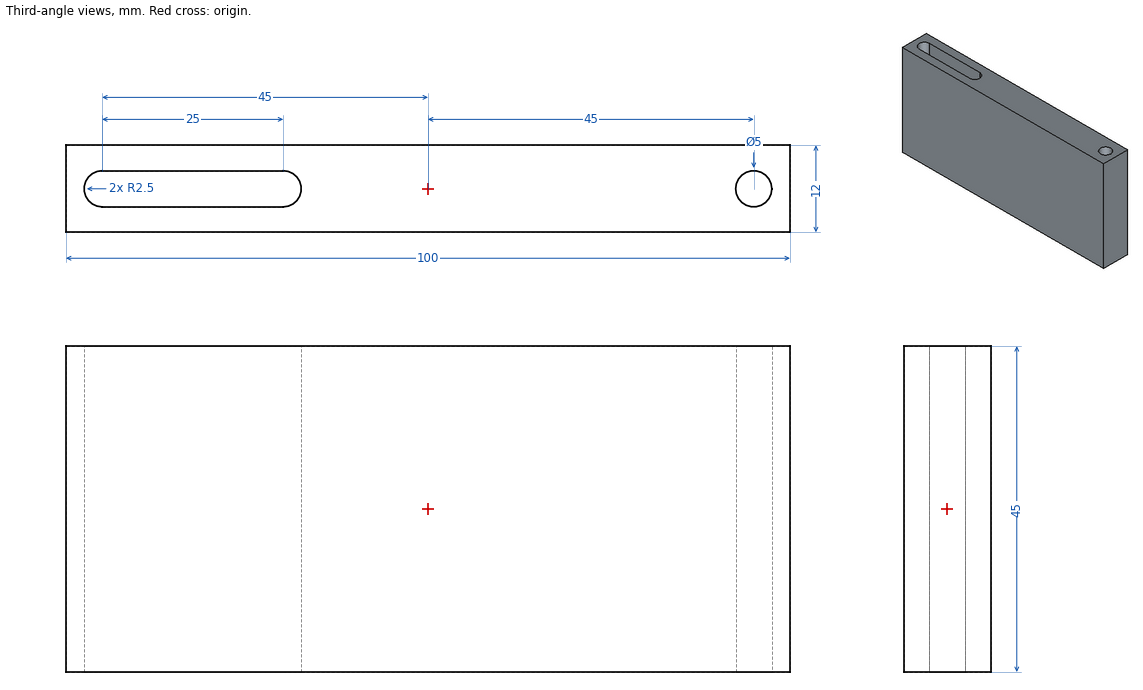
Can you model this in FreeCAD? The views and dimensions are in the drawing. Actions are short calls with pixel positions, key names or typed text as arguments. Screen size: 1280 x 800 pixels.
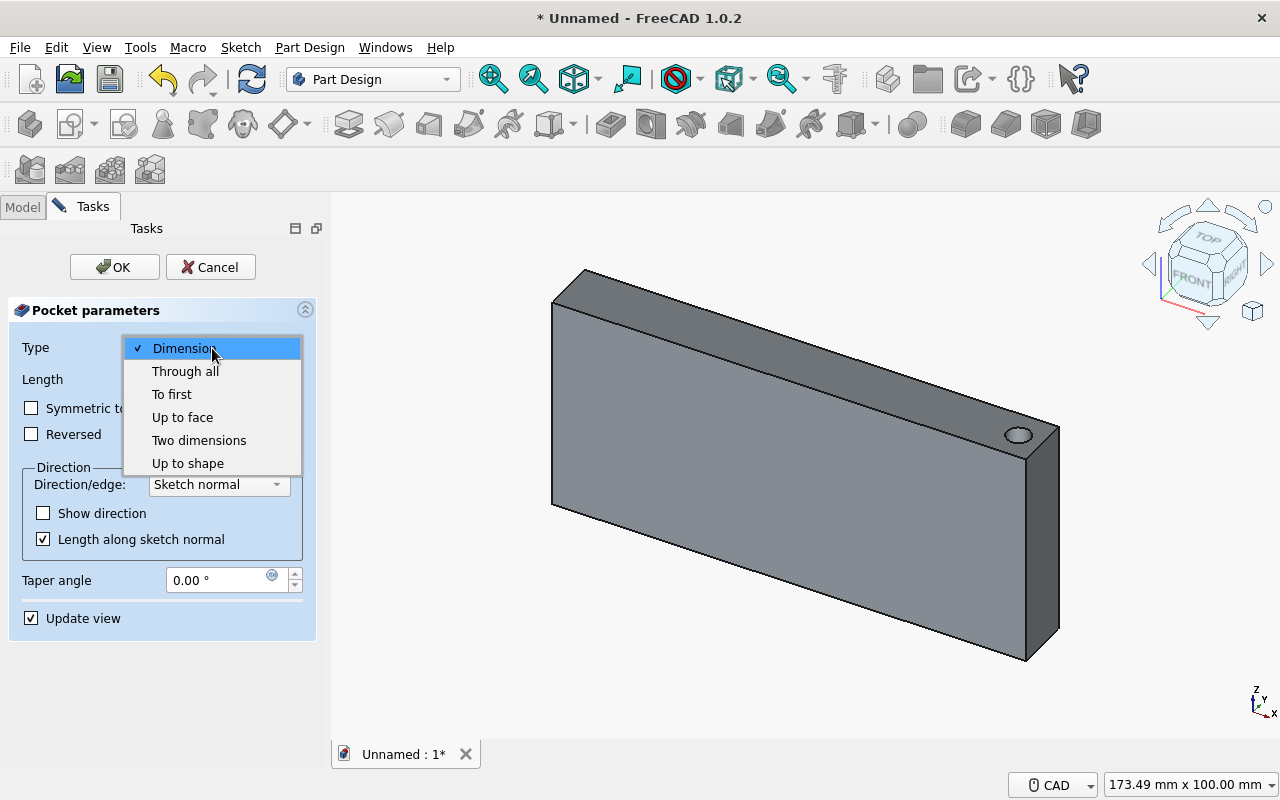
click(212, 394)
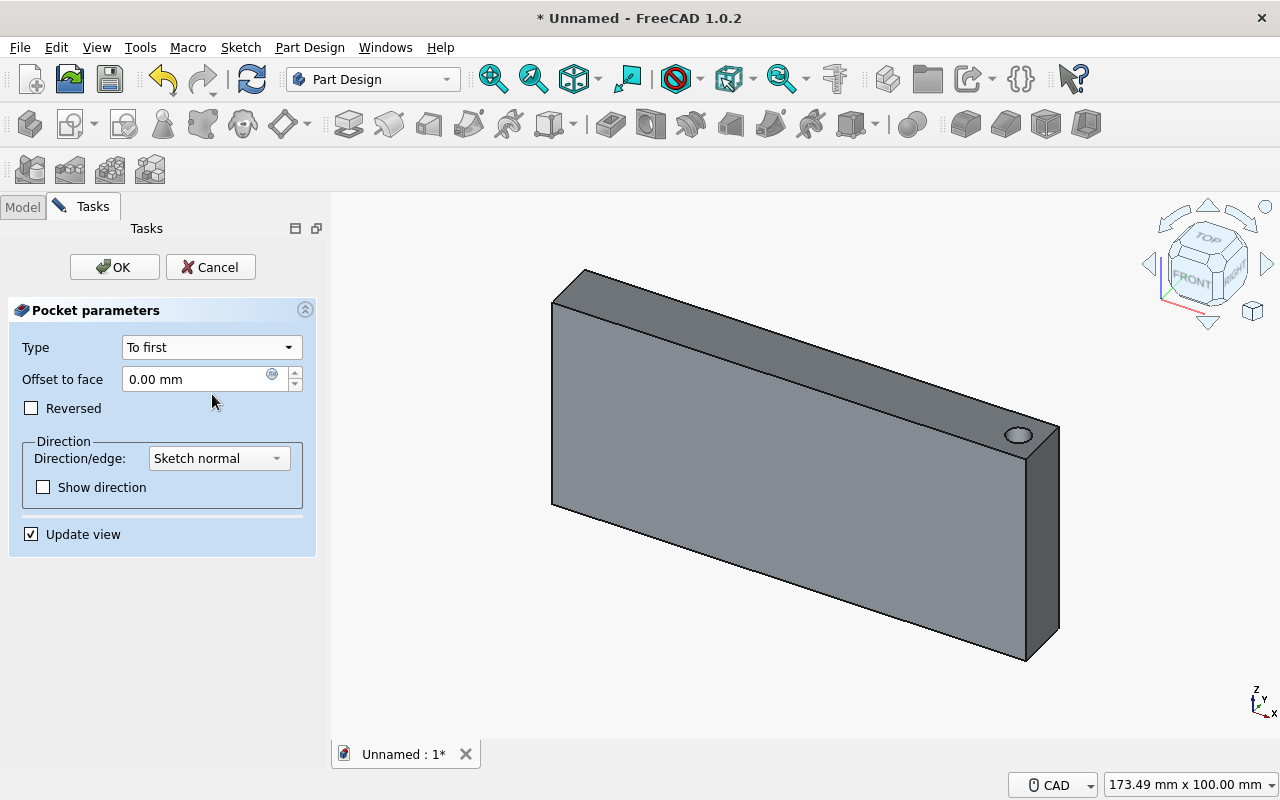
click(115, 267)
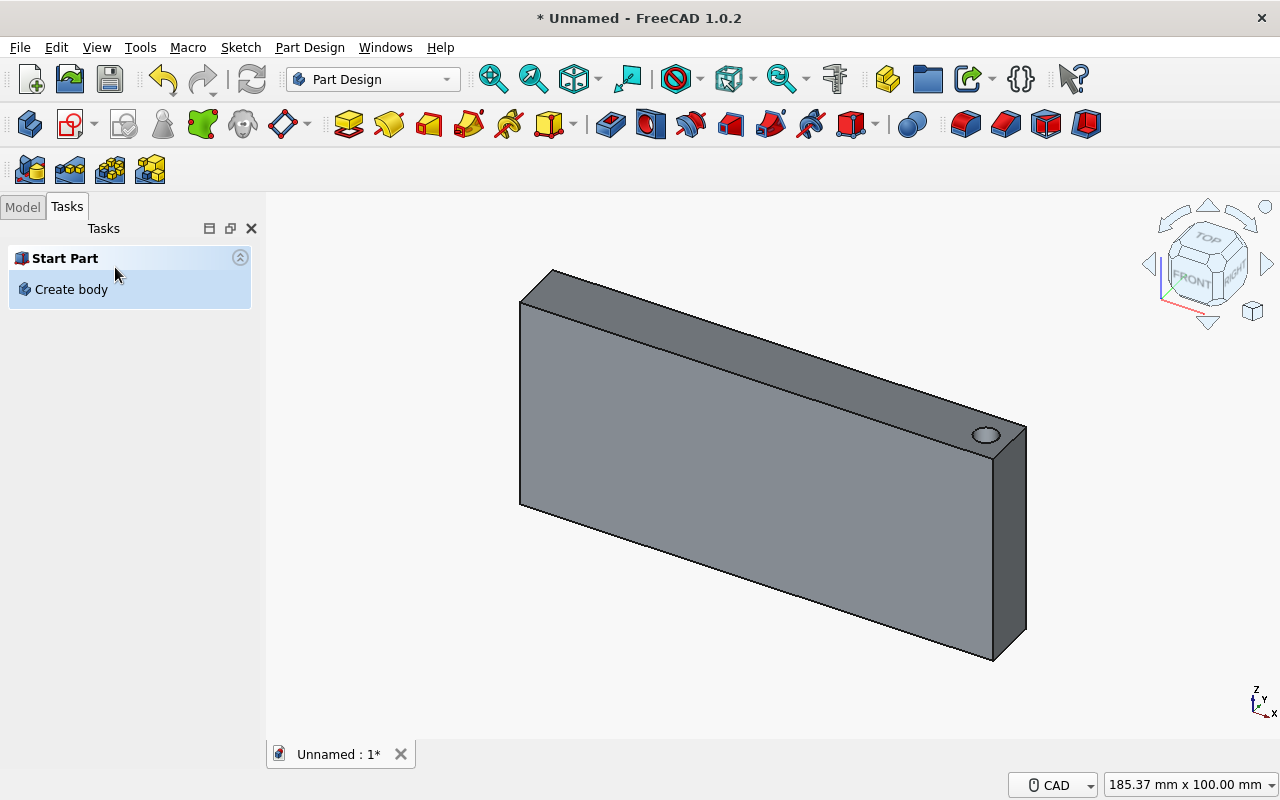
click(908, 409)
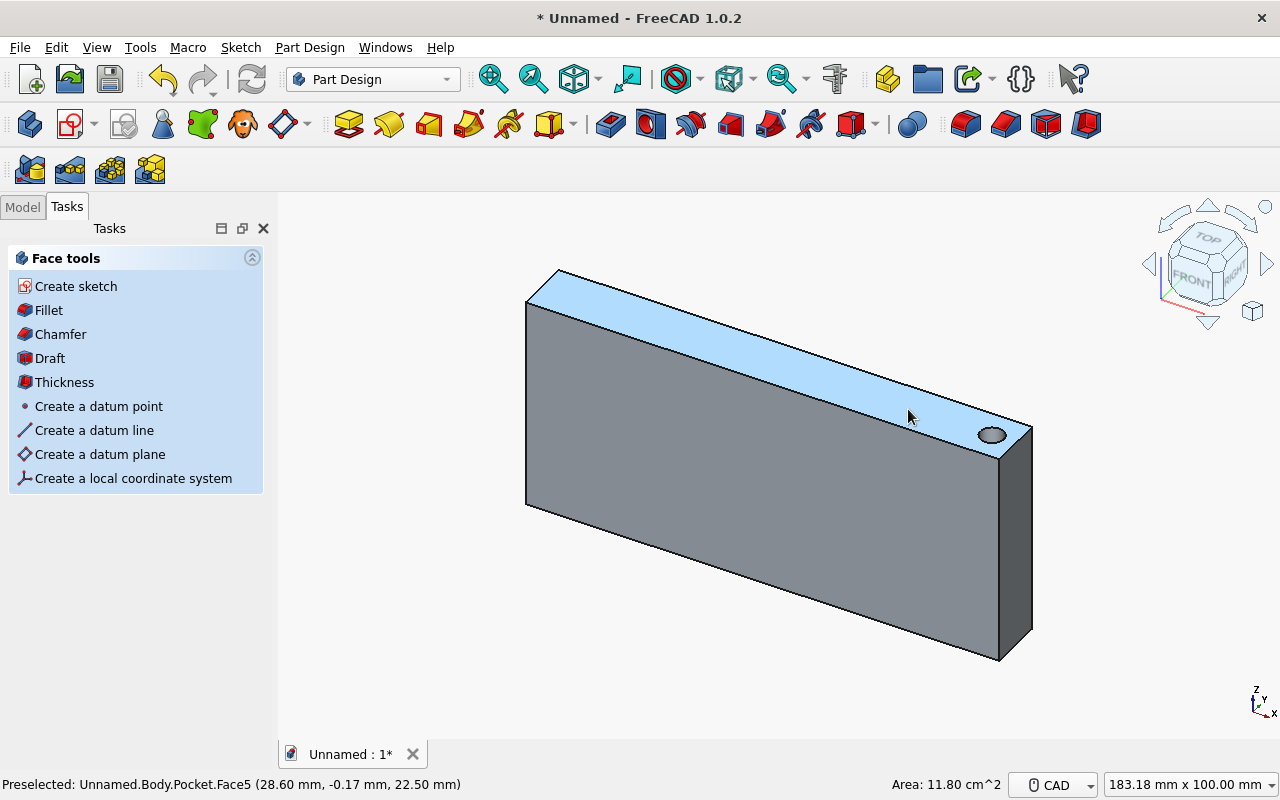
click(70, 124)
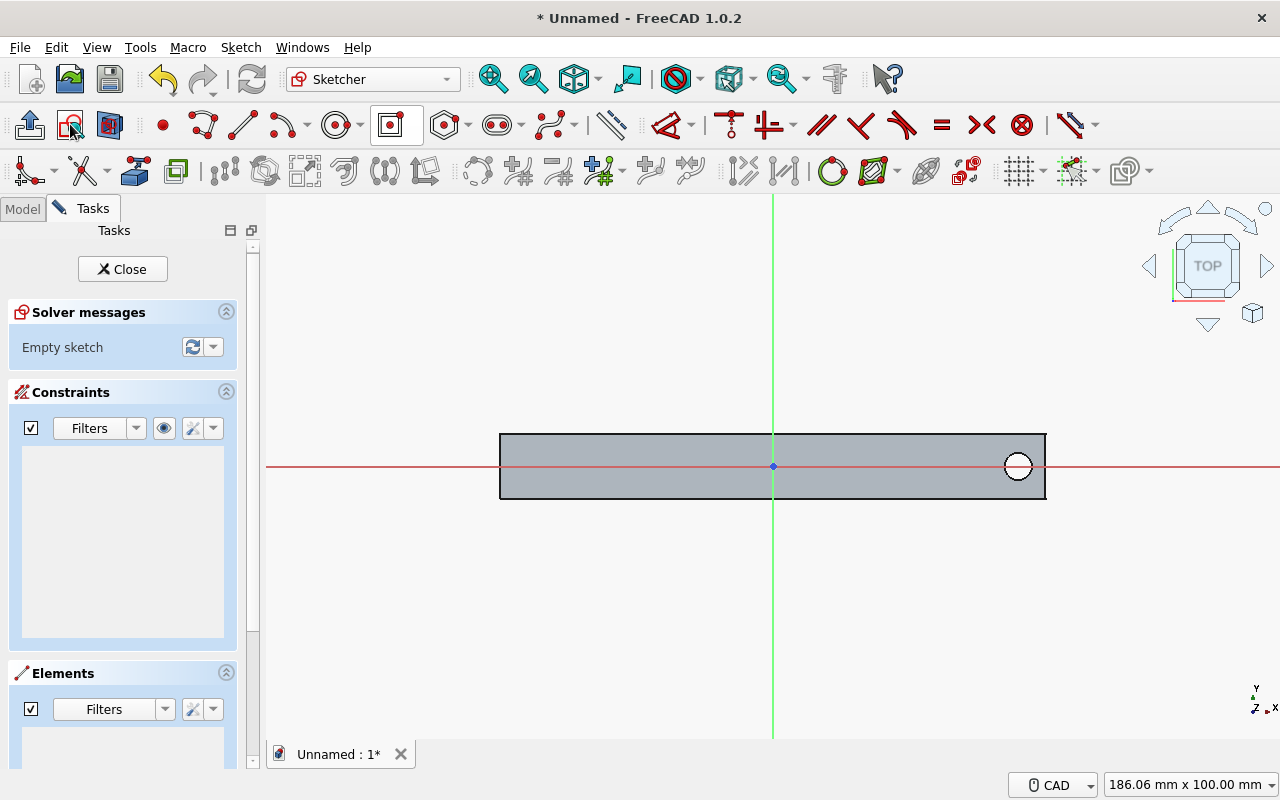
scroll(594, 467, up, 4)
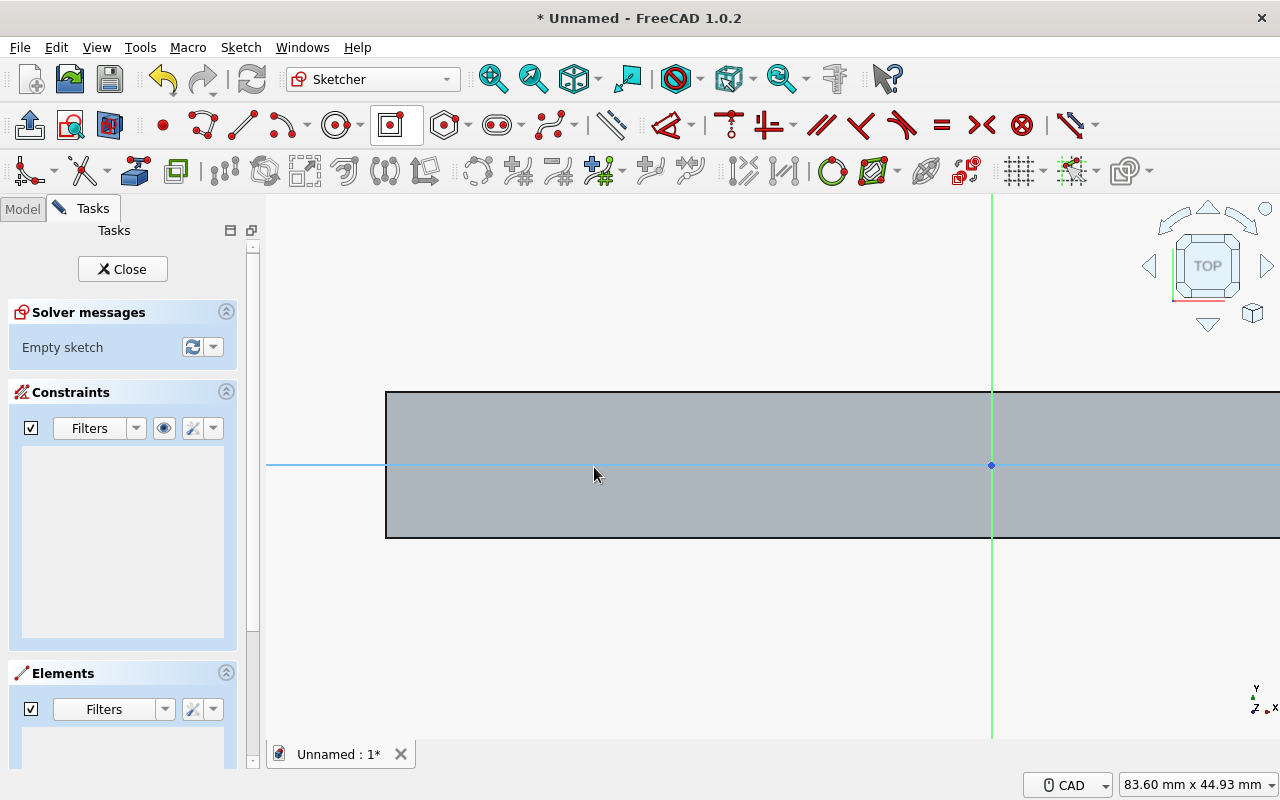
click(498, 126)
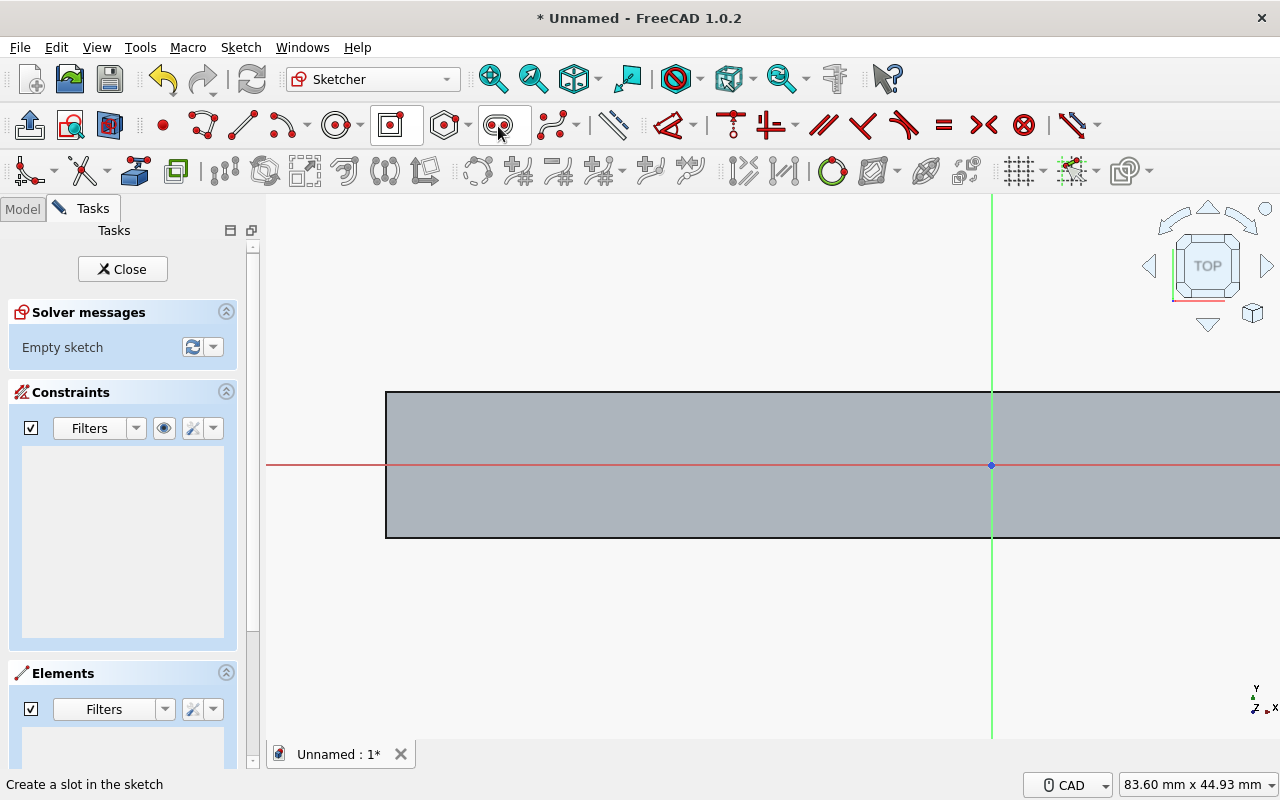
click(446, 465)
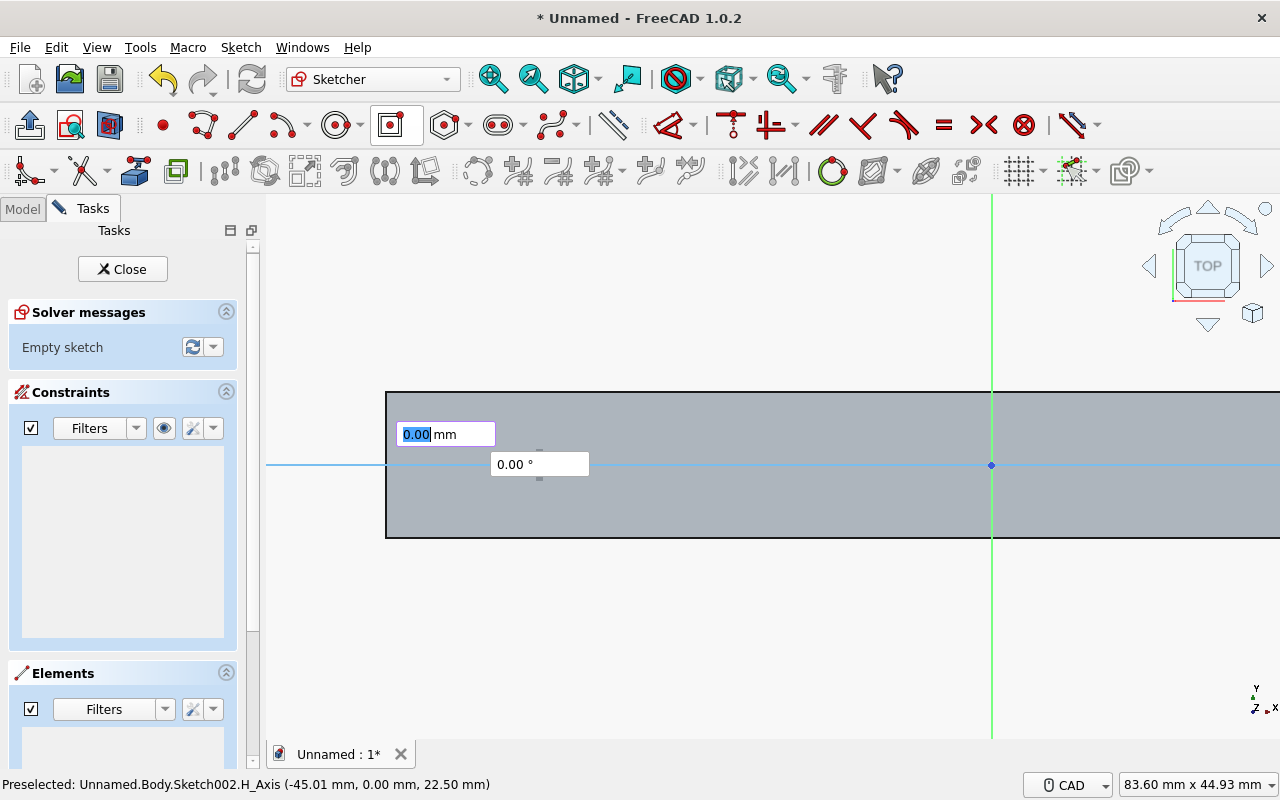
click(749, 456)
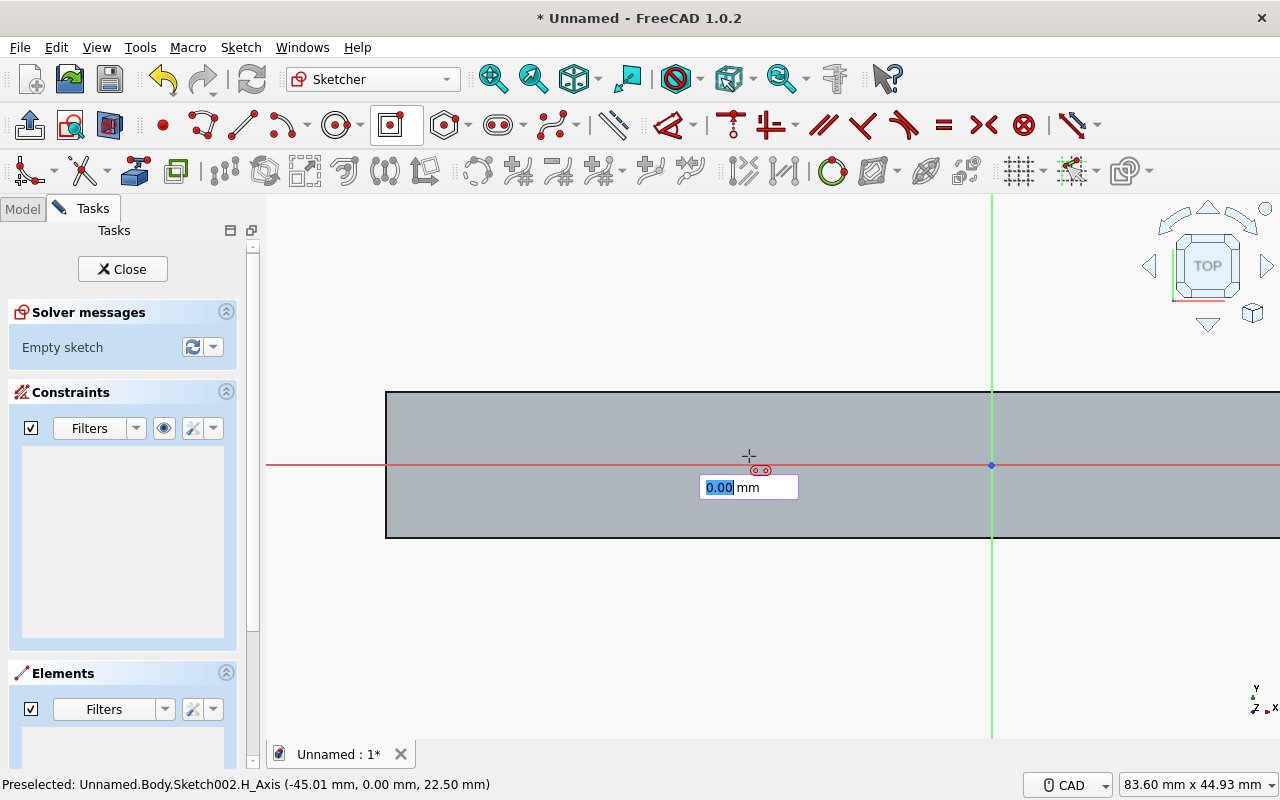
click(598, 435)
key(Escape)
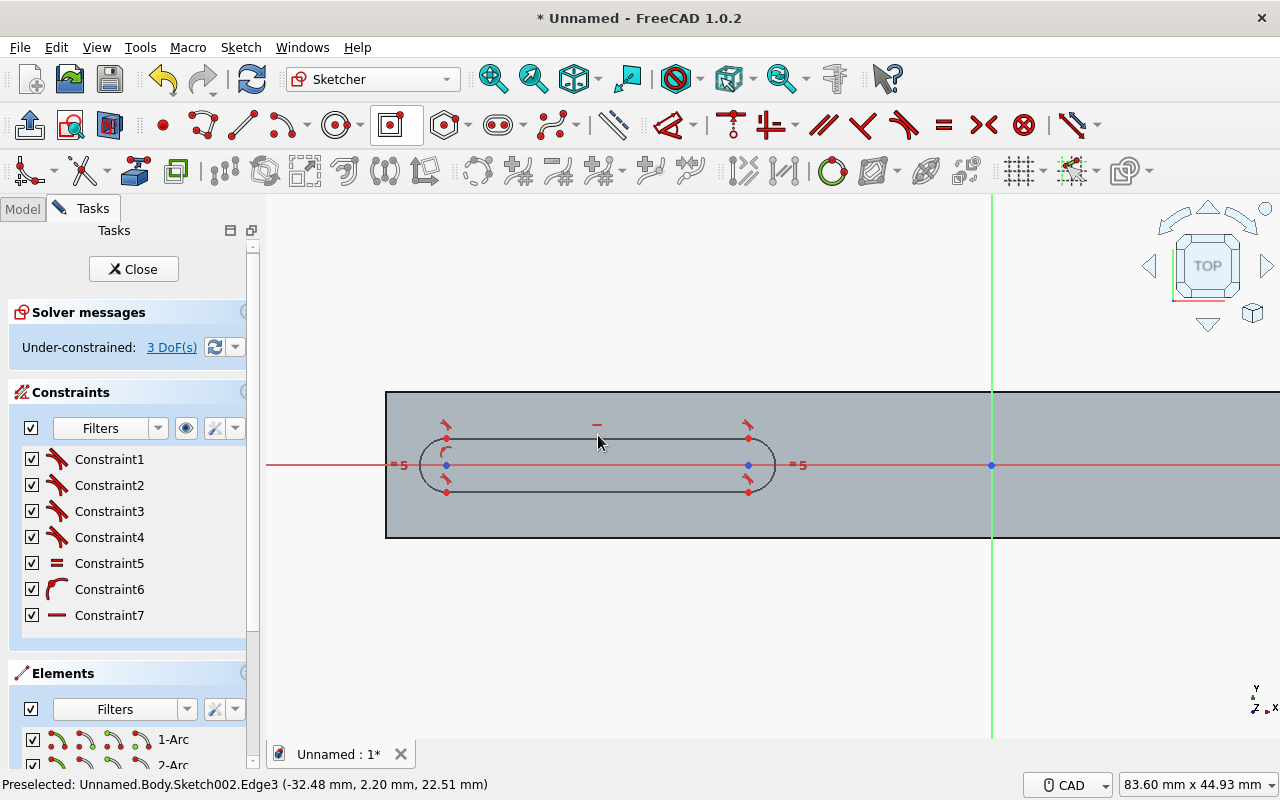
click(668, 126)